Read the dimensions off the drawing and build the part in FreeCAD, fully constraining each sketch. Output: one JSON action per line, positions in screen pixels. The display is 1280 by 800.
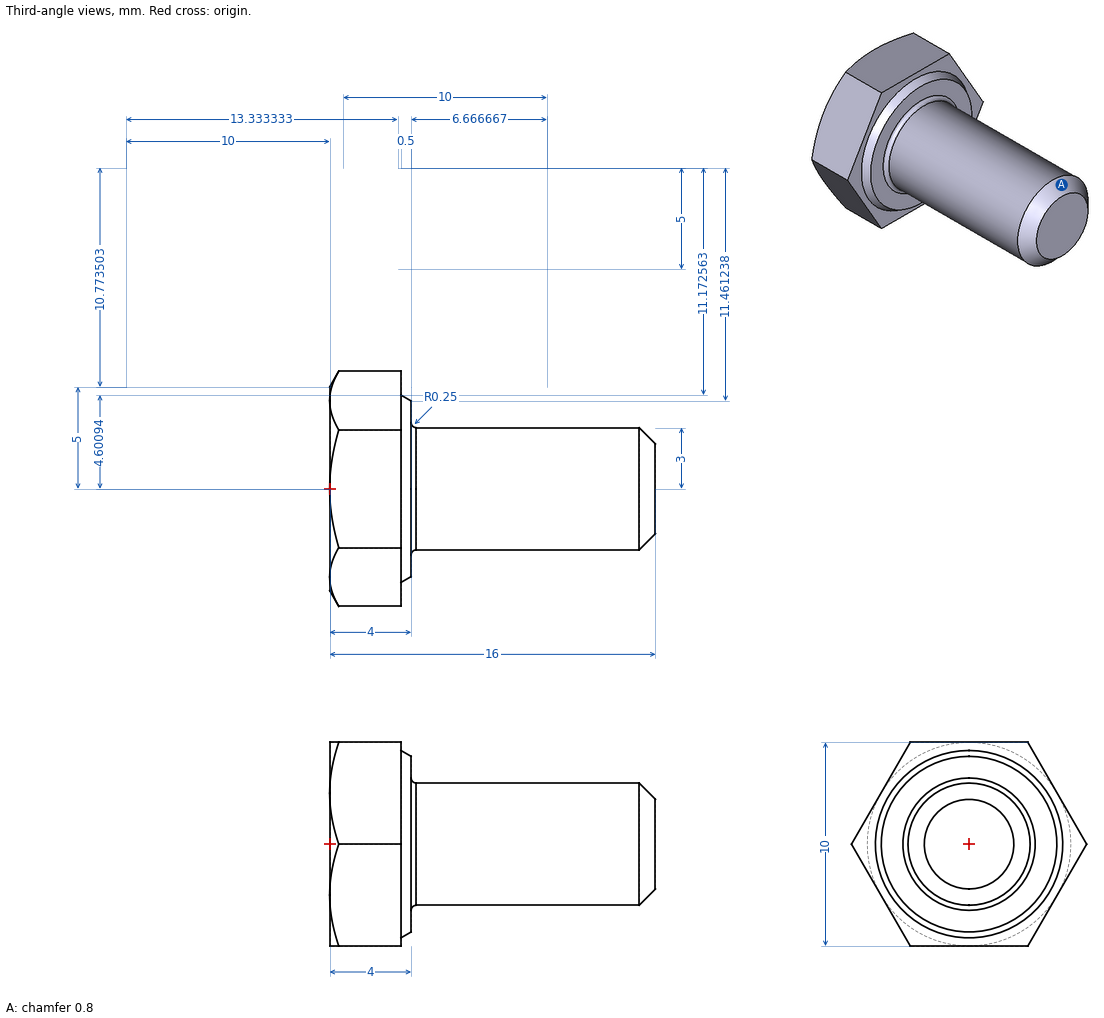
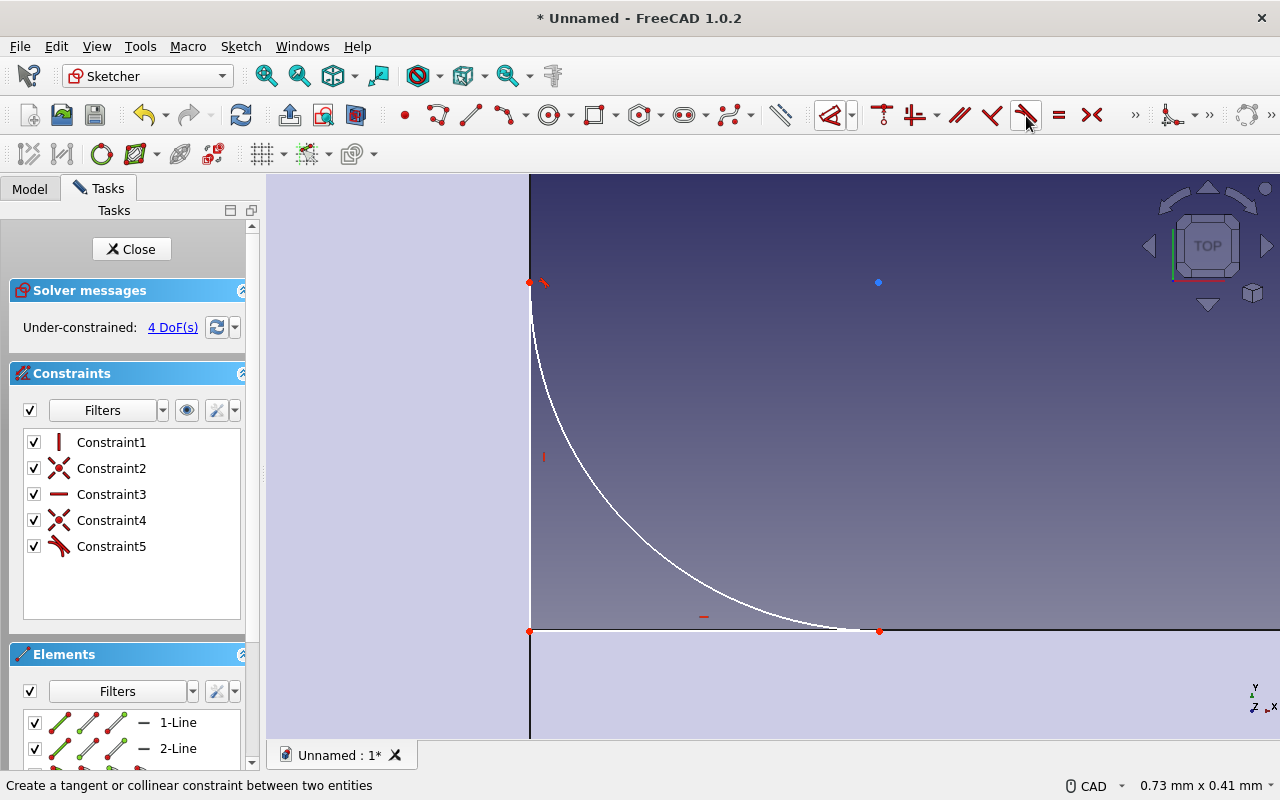
{"action": "left_click", "coordinate": [635, 631]}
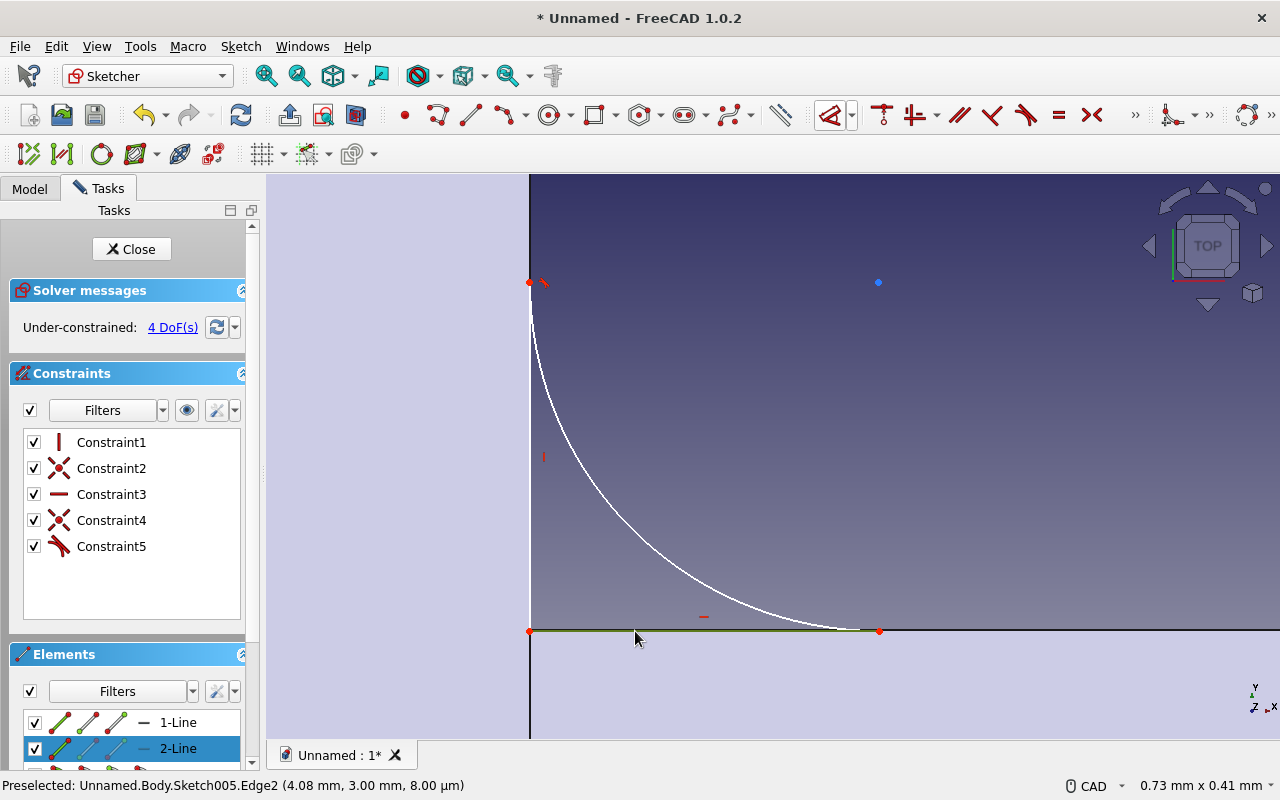
{"action": "left_click", "coordinate": [568, 441]}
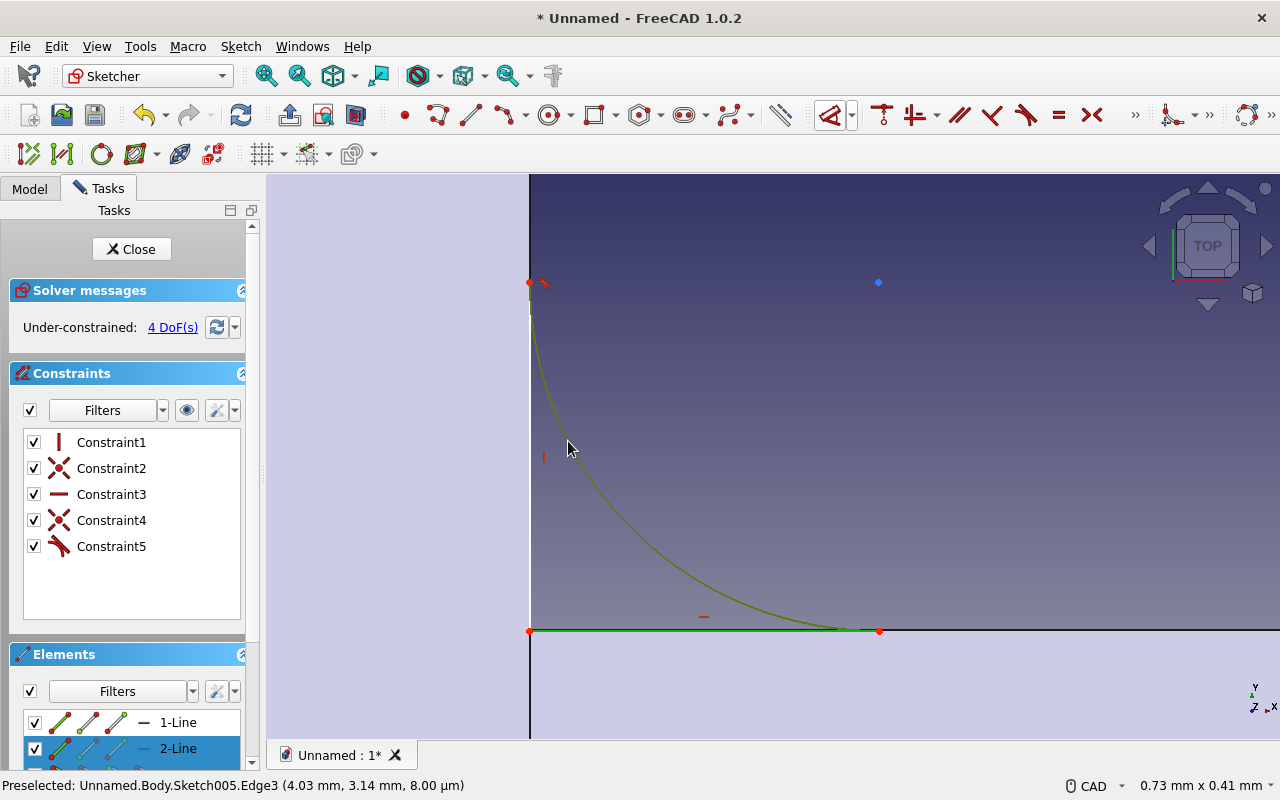
{"action": "left_click", "coordinate": [1026, 116]}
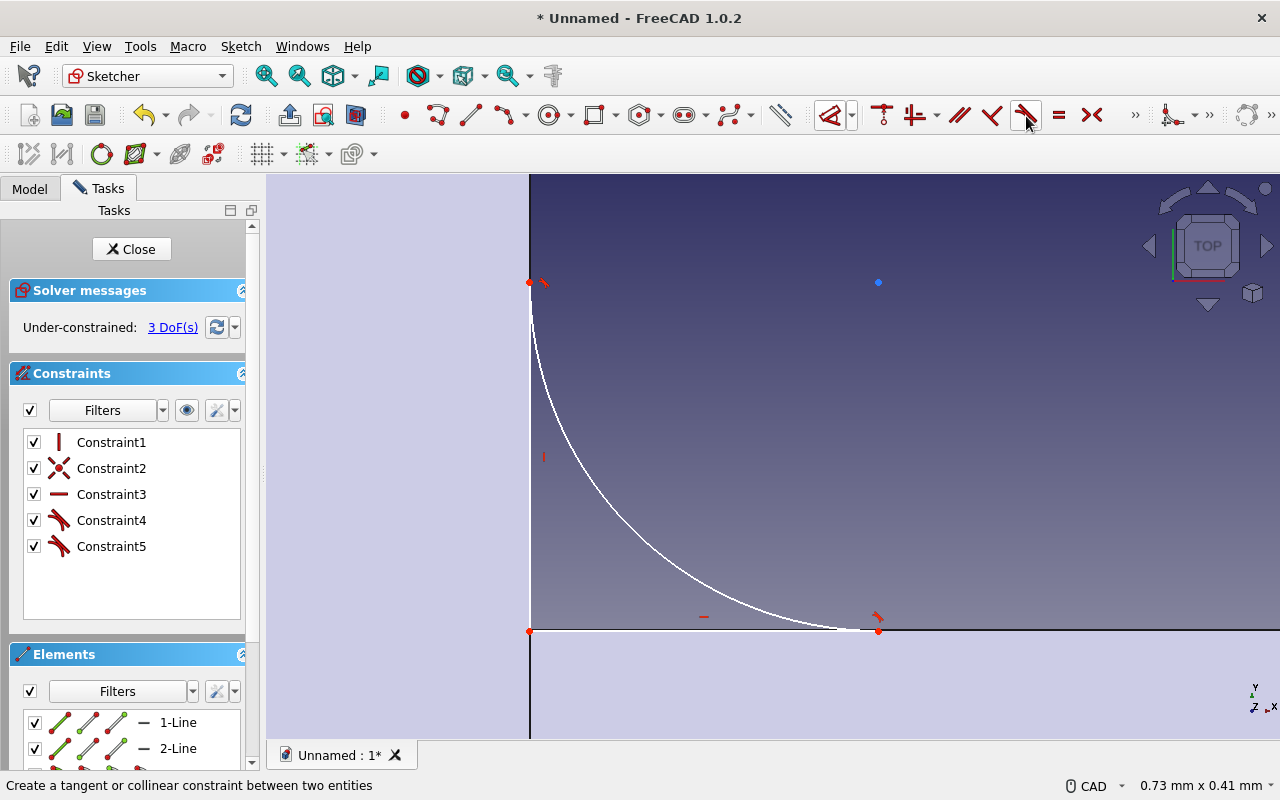
{"action": "left_click", "coordinate": [568, 441]}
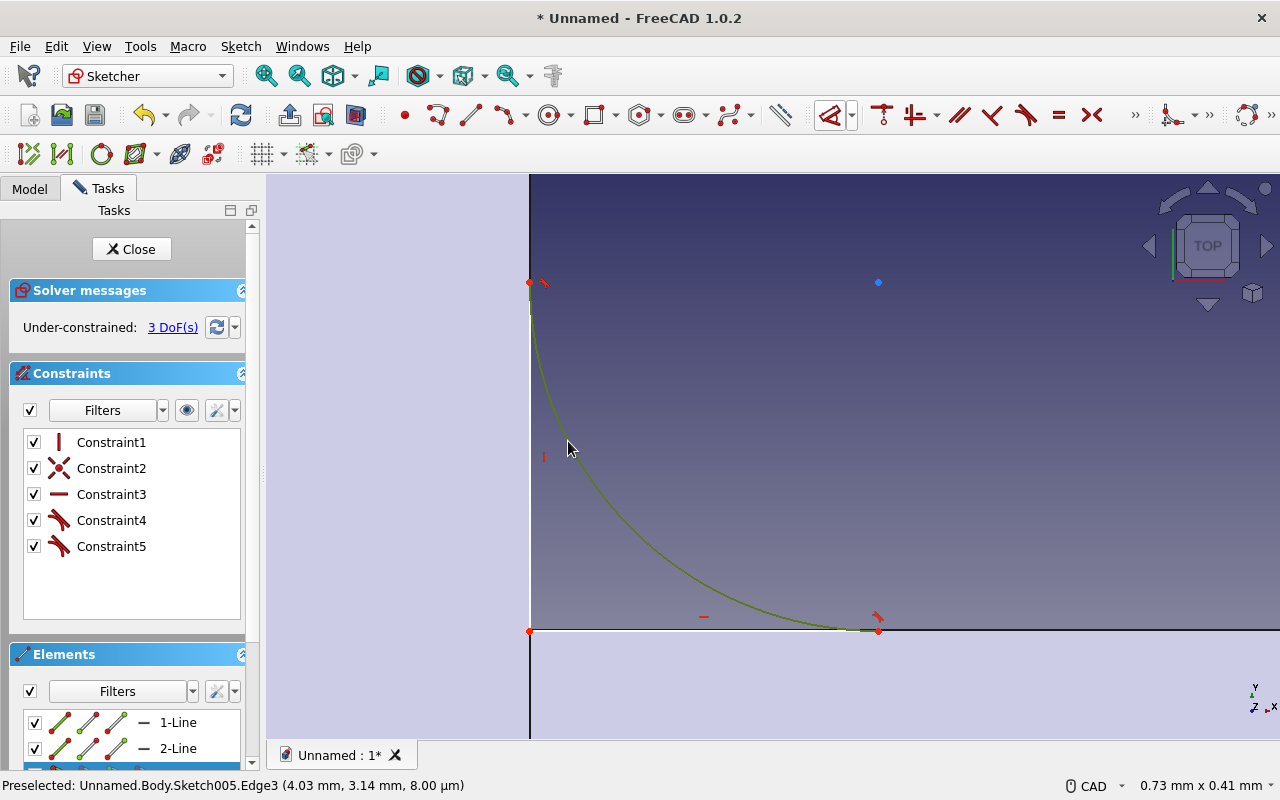
{"action": "left_click", "coordinate": [852, 116]}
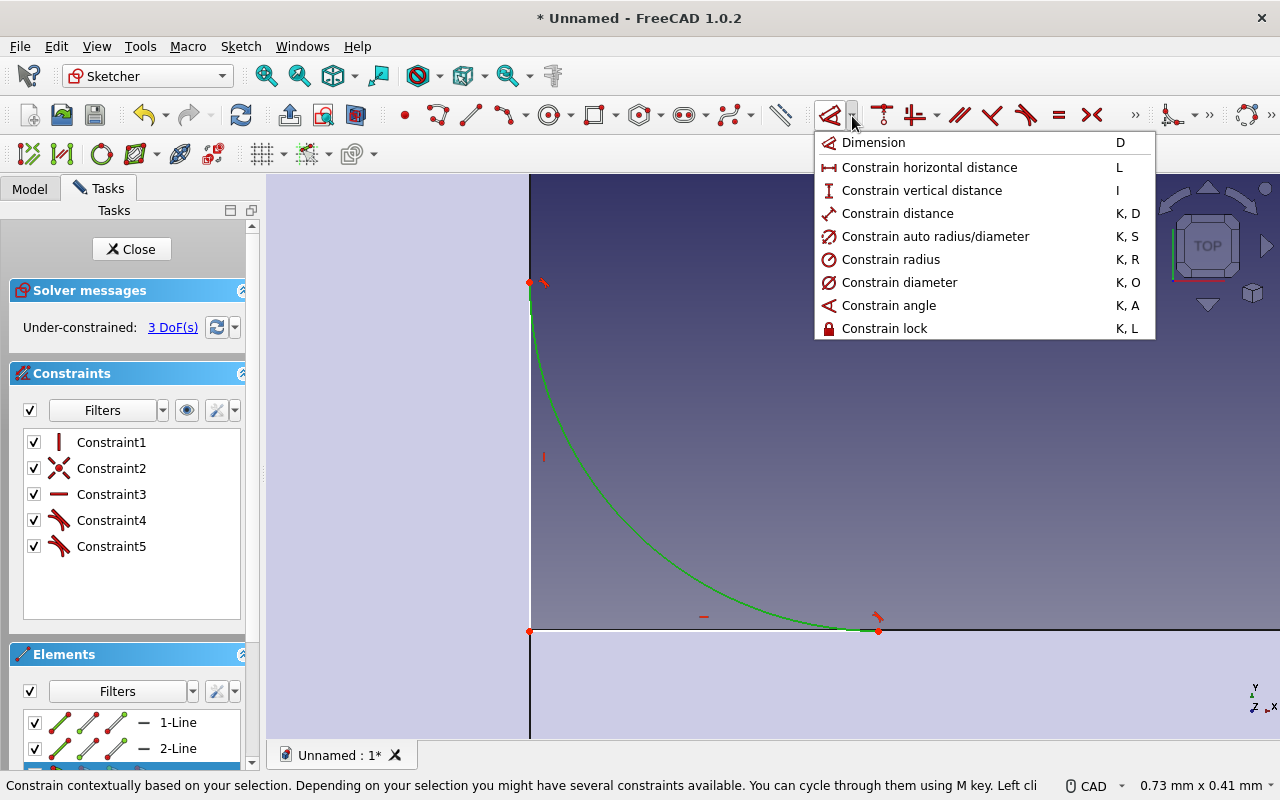
{"action": "left_click", "coordinate": [985, 260]}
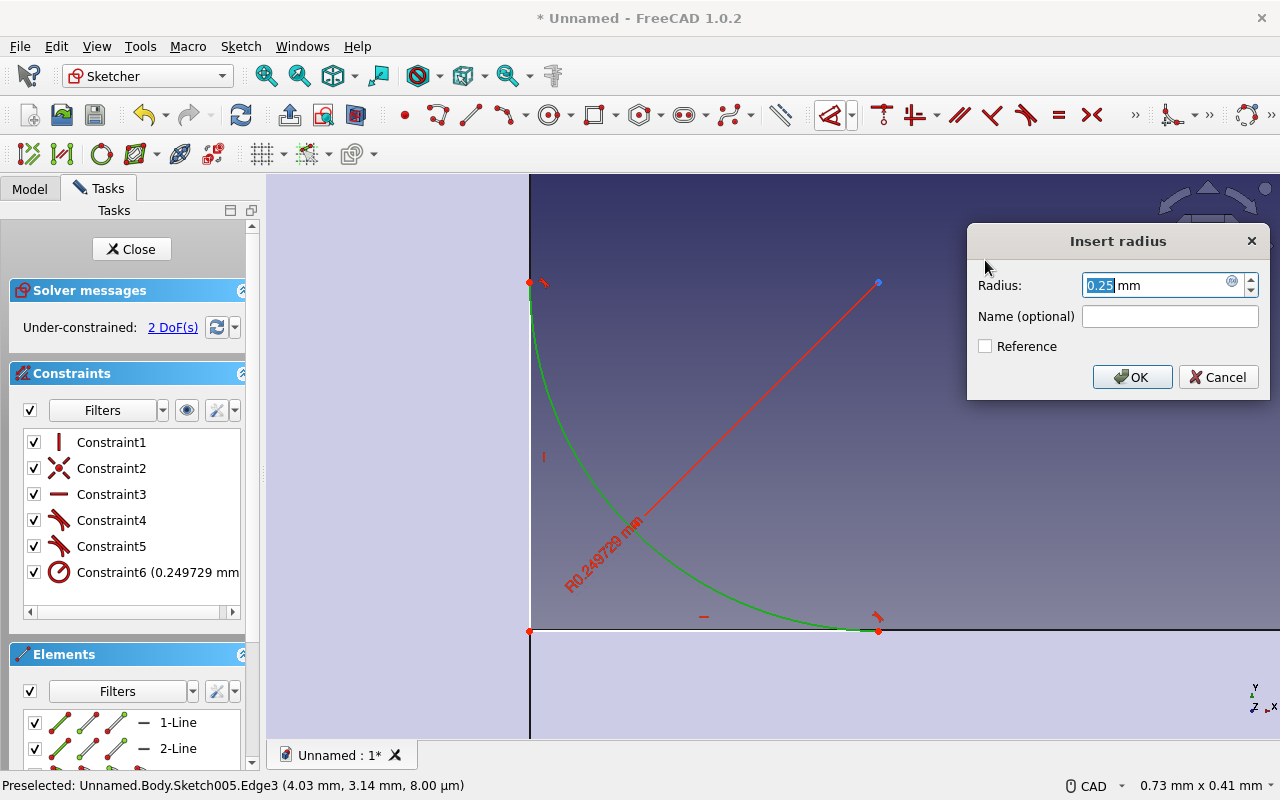
{"action": "type", "text": "0.25"}
{"action": "key", "text": "Return"}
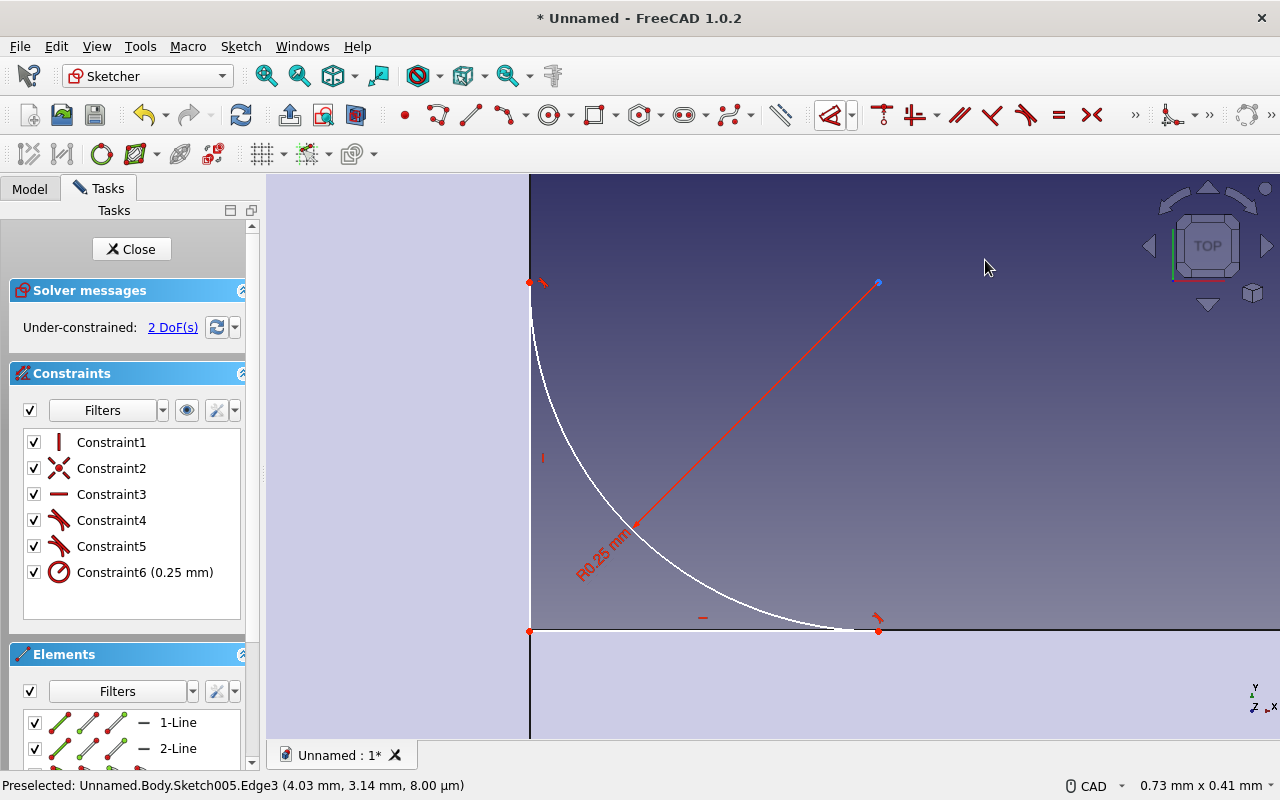
{"action": "left_click", "coordinate": [530, 283]}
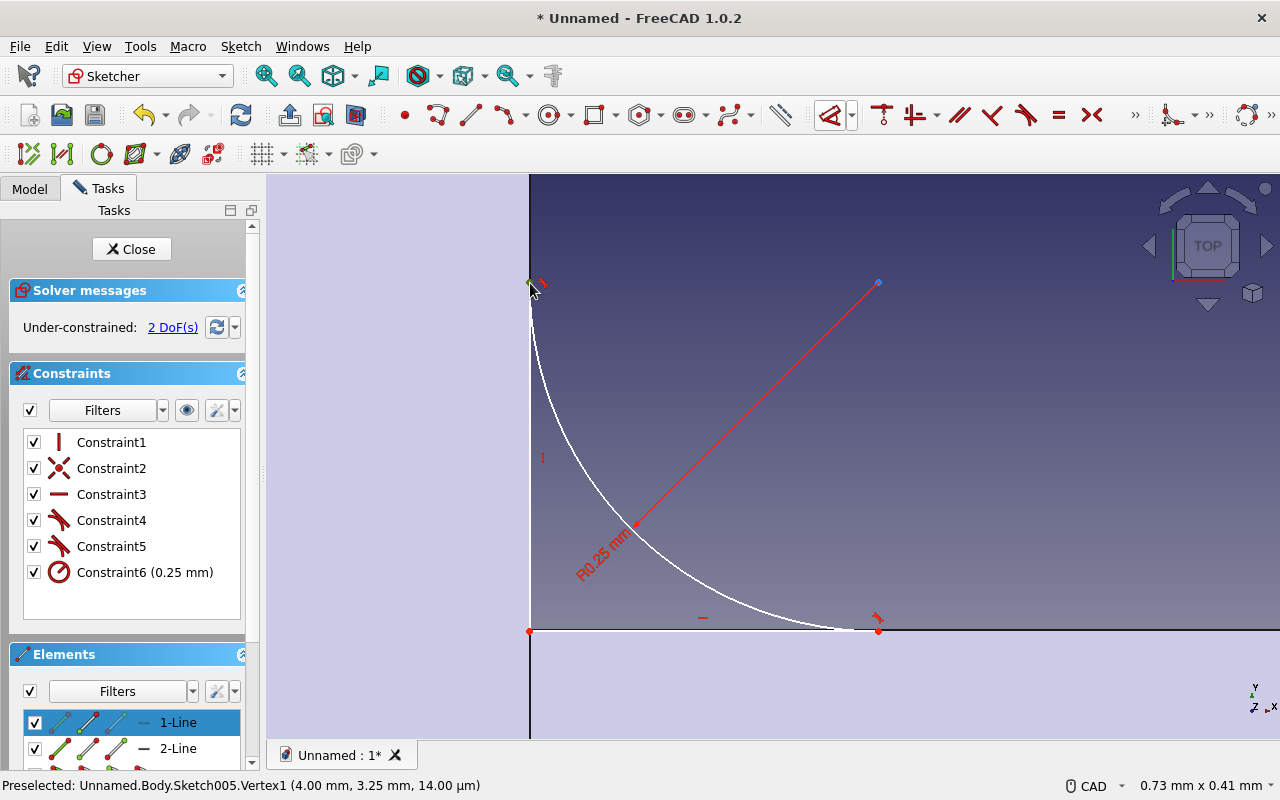
{"action": "key", "text": "l"}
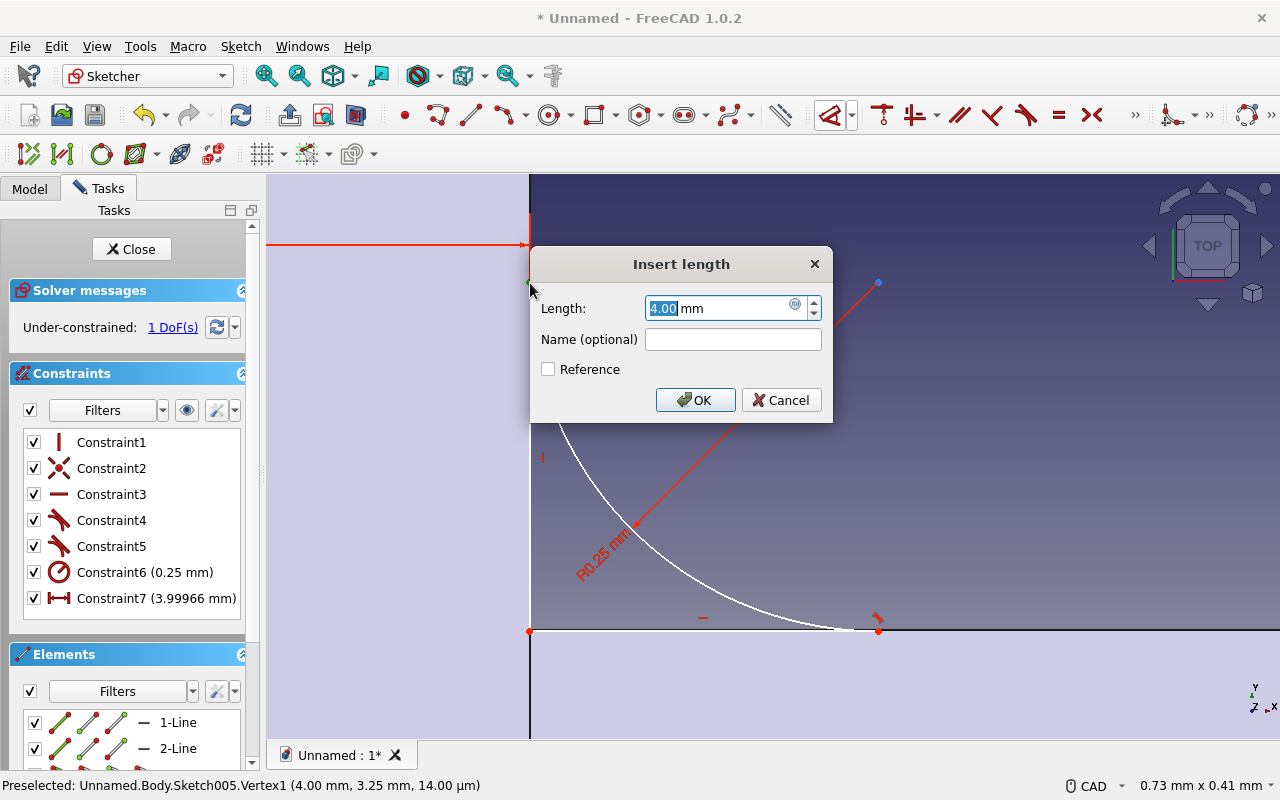
{"action": "type", "text": "4"}
{"action": "key", "text": "Return"}